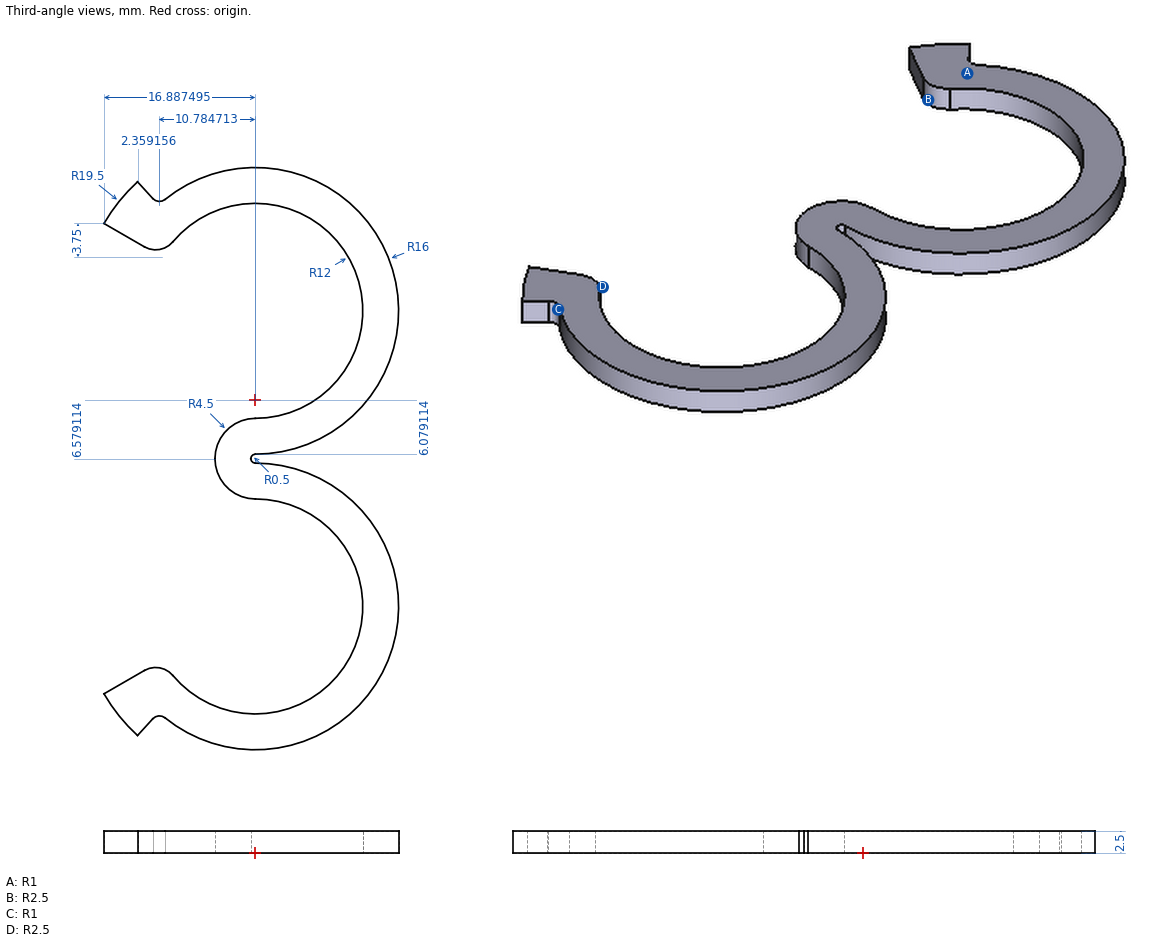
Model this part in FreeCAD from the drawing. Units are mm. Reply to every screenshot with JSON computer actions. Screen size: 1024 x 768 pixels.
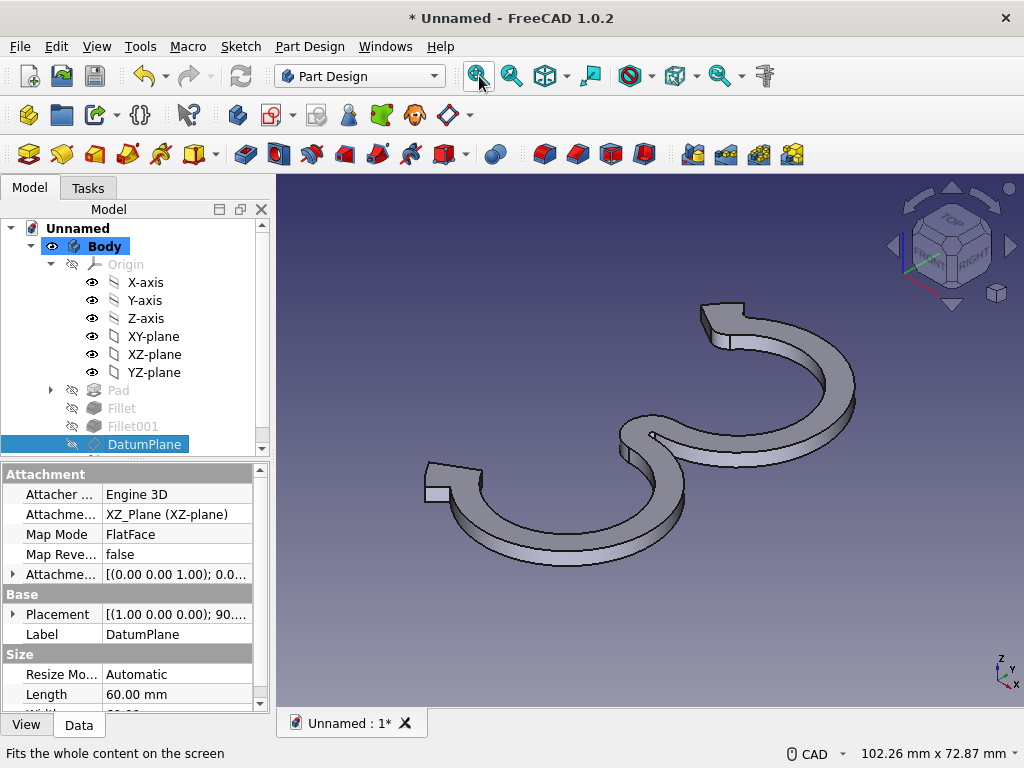
{"action": "key", "text": "2"}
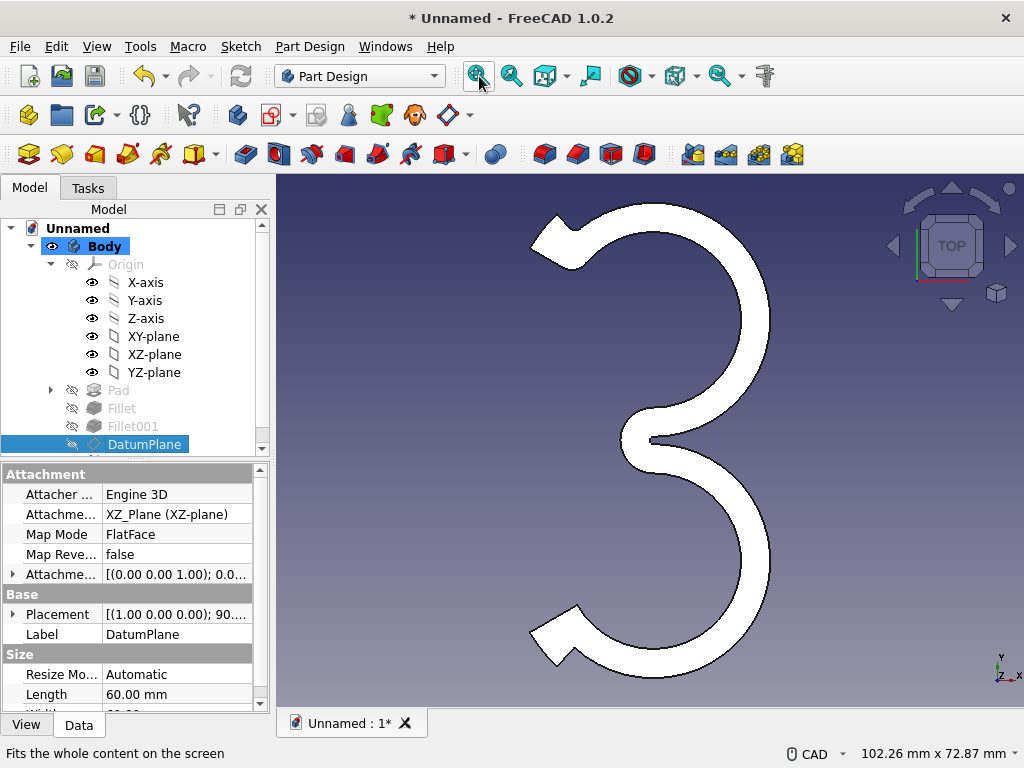
{"action": "scroll", "coordinate": [574, 647], "scroll_direction": "up", "scroll_amount": 4}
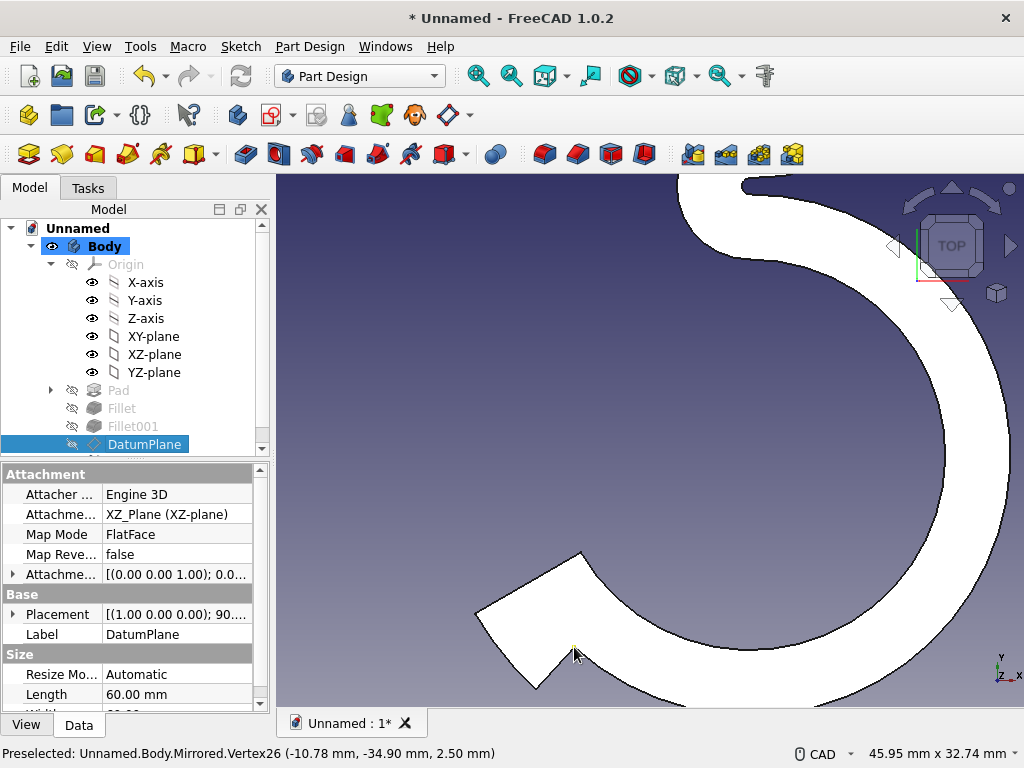
{"action": "left_click", "coordinate": [479, 76]}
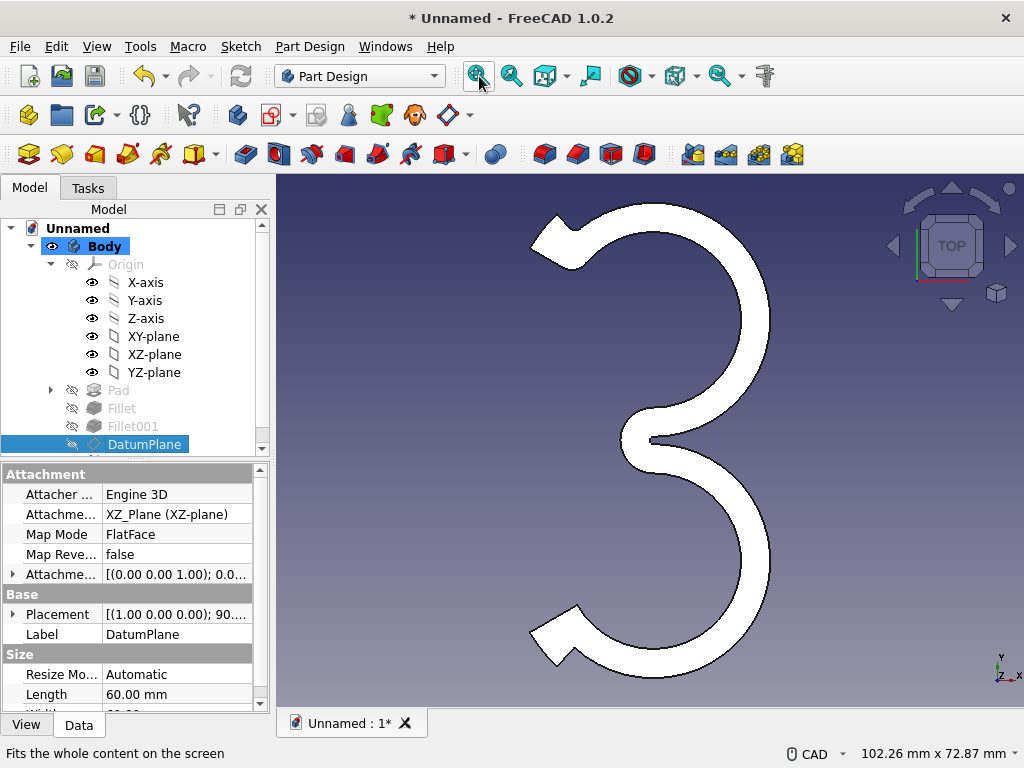
{"action": "key", "text": "0"}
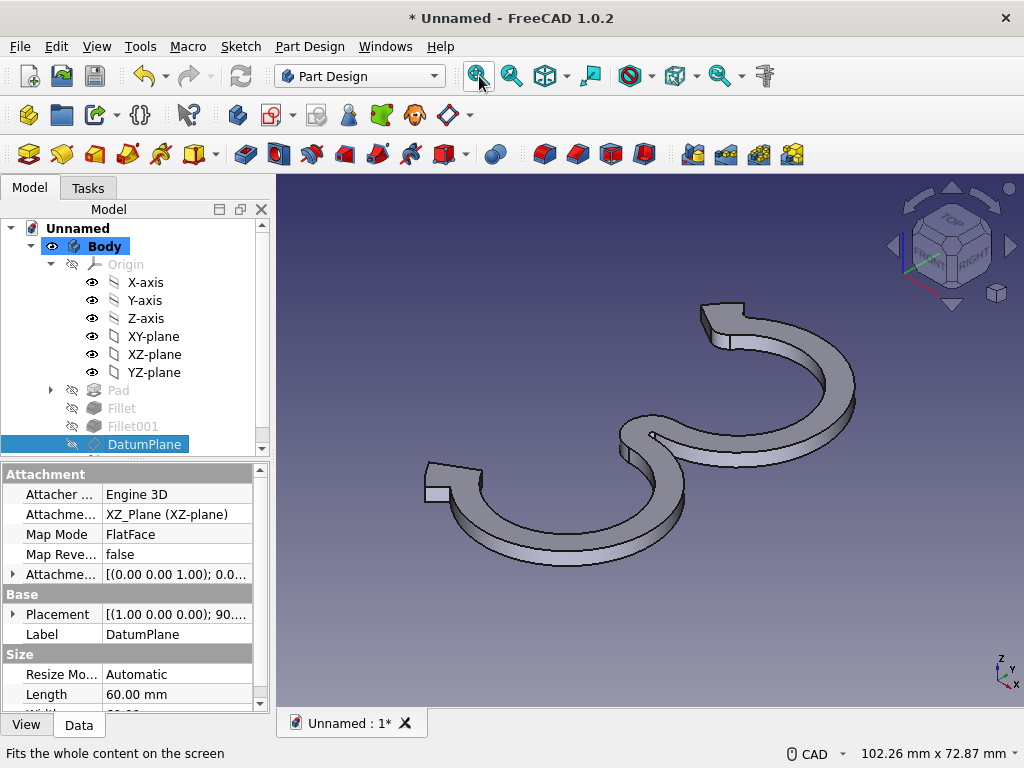
{"action": "scroll", "coordinate": [450, 493], "scroll_direction": "up", "scroll_amount": 4}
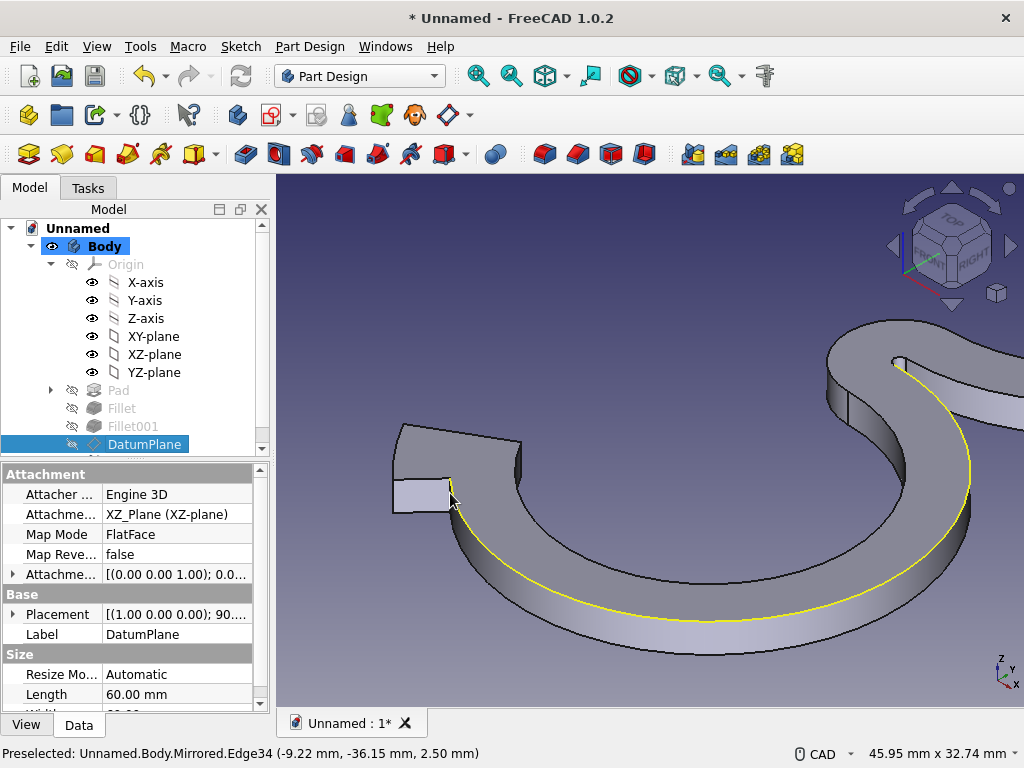
{"action": "left_click", "coordinate": [479, 76]}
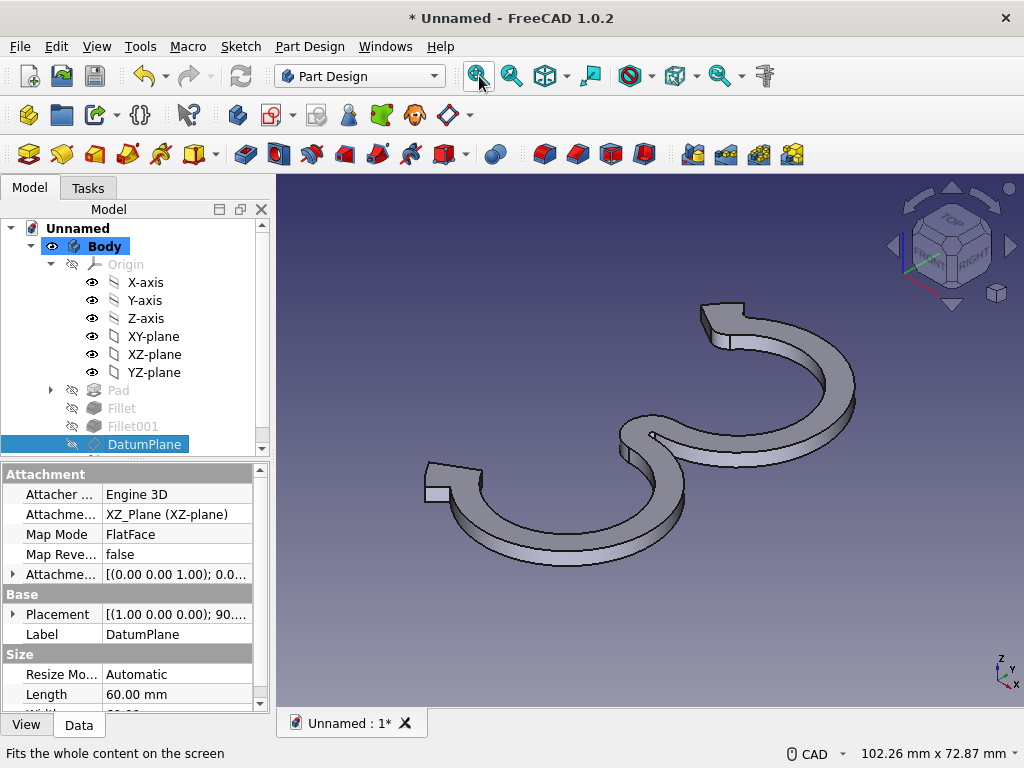
{"action": "key", "text": "1"}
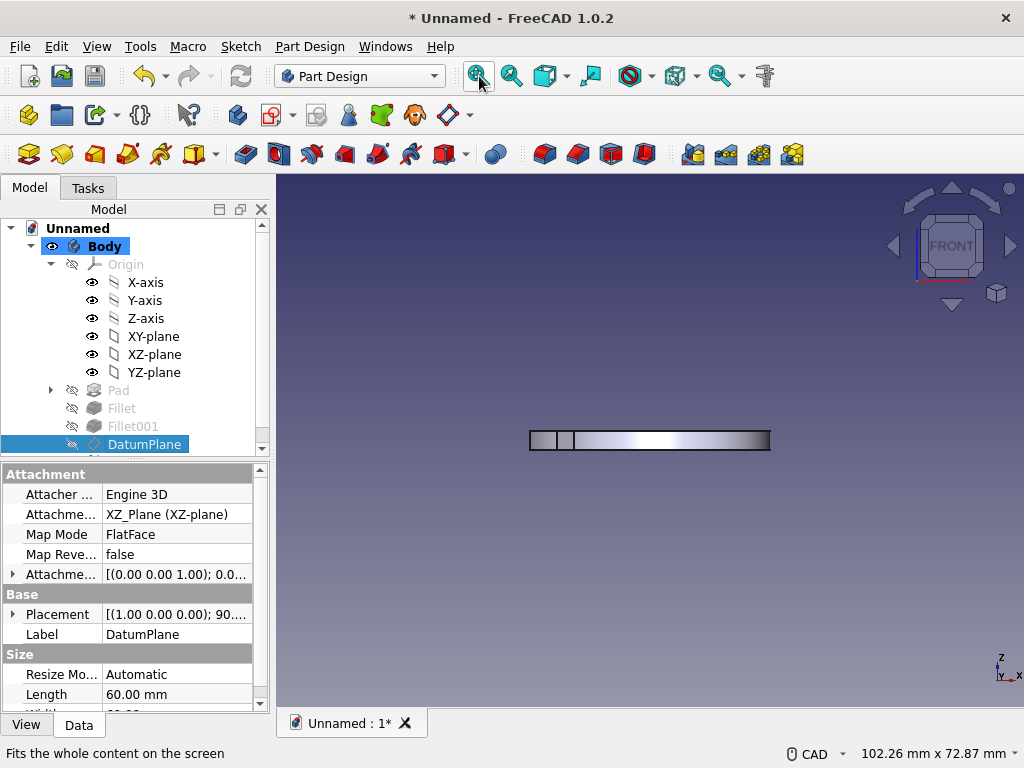
{"action": "left_click", "coordinate": [479, 76]}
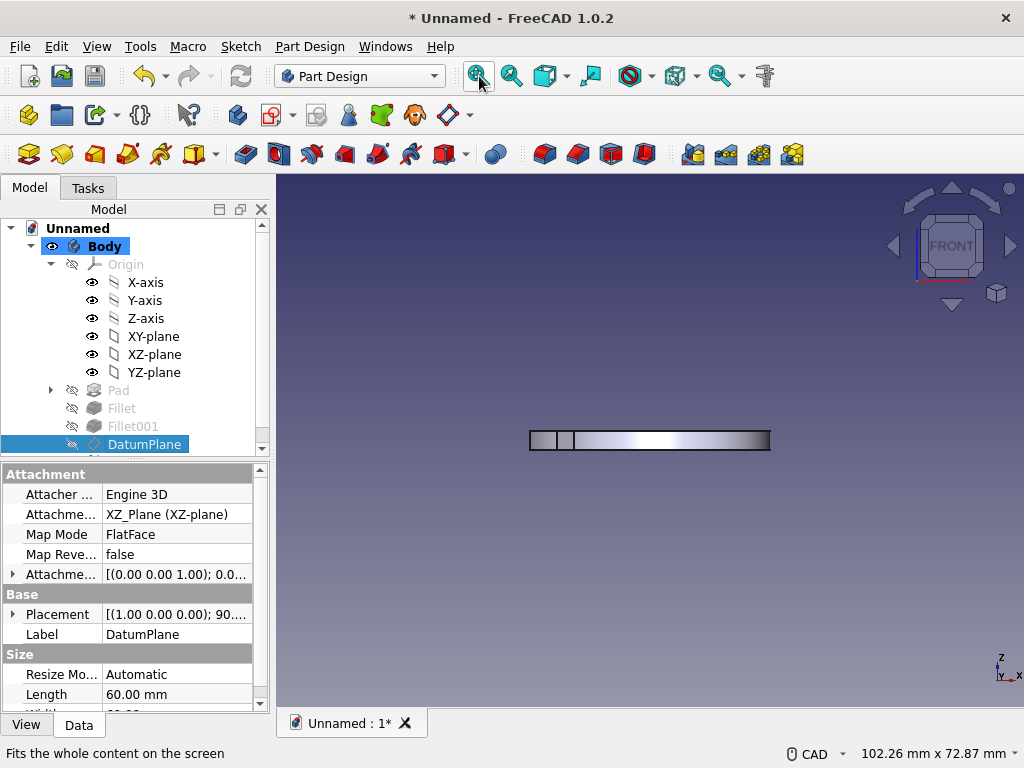
{"action": "scroll", "coordinate": [574, 440], "scroll_direction": "up", "scroll_amount": 4}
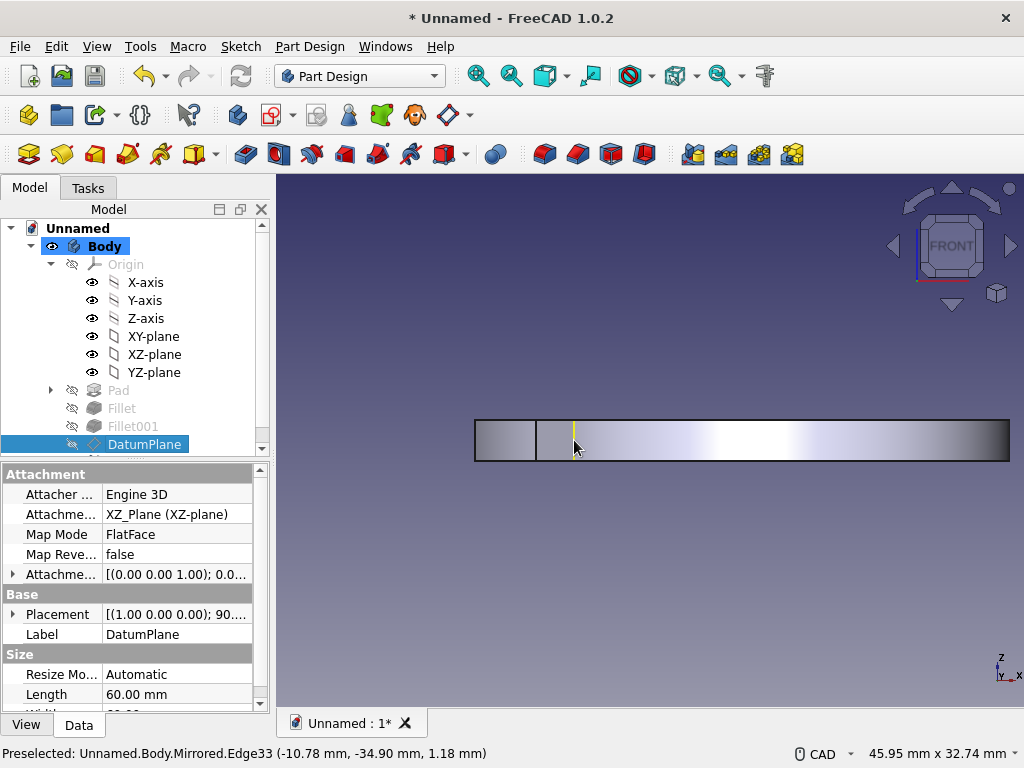
{"action": "left_click", "coordinate": [479, 76]}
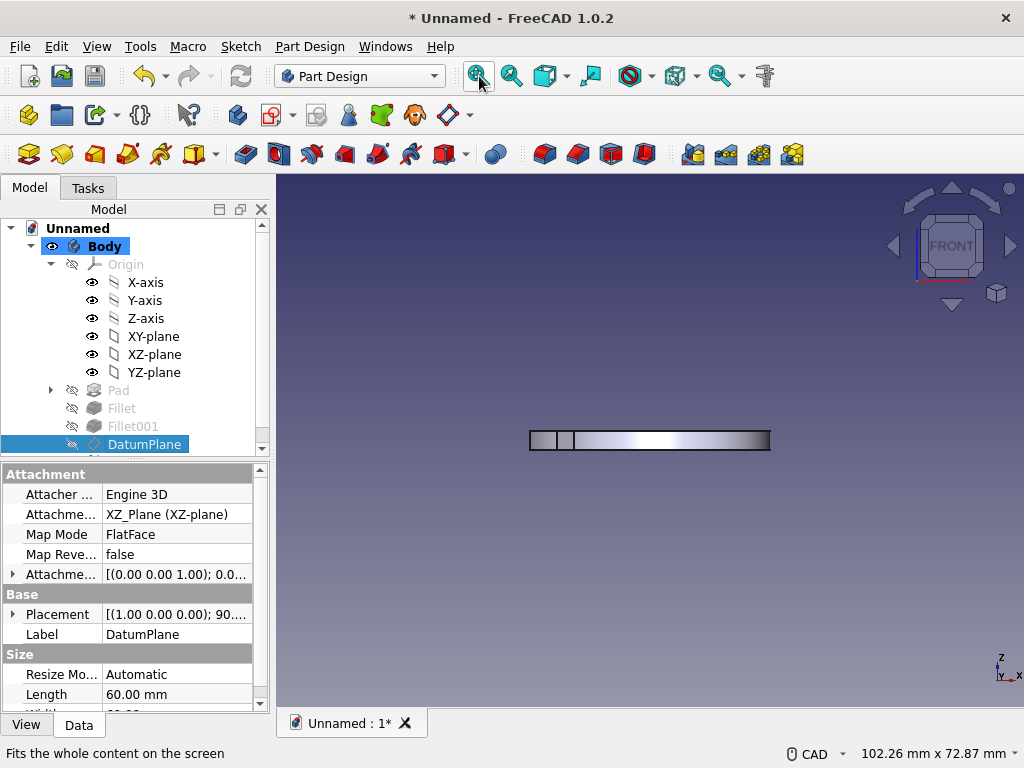
{"action": "key", "text": "3"}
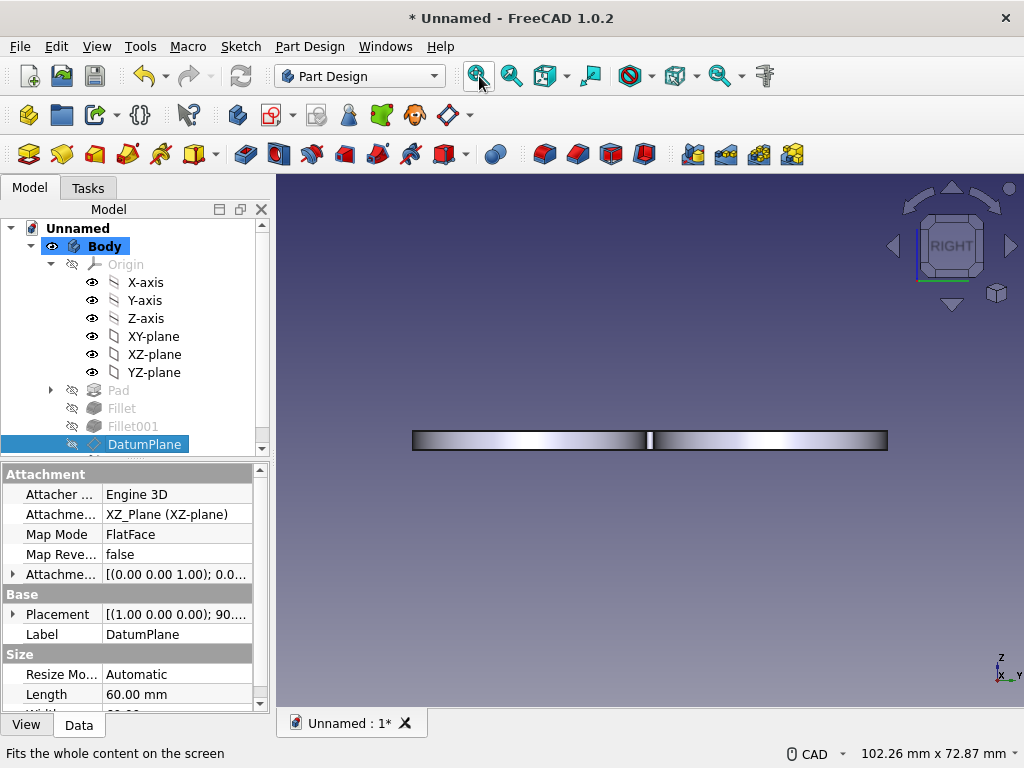
{"action": "scroll", "coordinate": [443, 439], "scroll_direction": "up", "scroll_amount": 4}